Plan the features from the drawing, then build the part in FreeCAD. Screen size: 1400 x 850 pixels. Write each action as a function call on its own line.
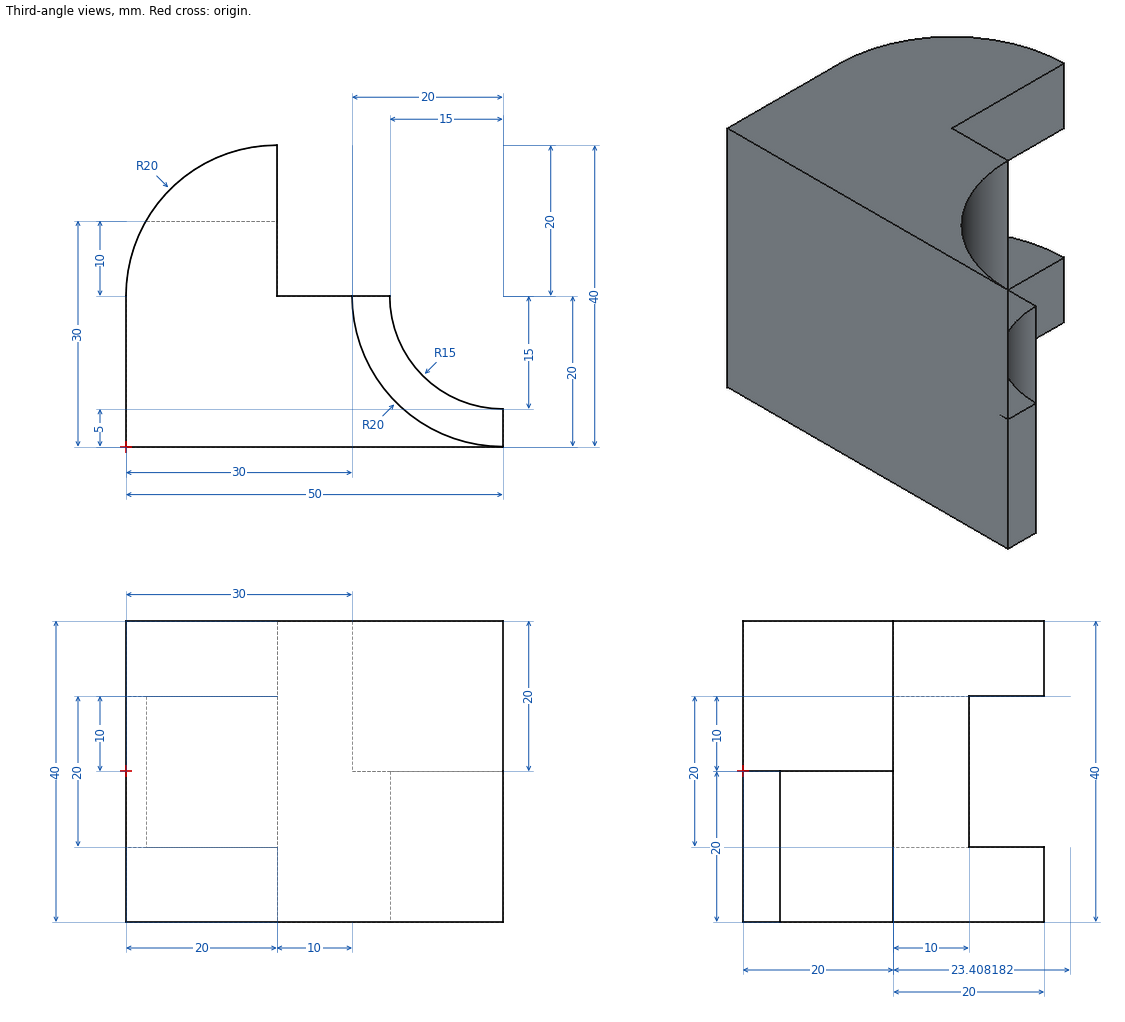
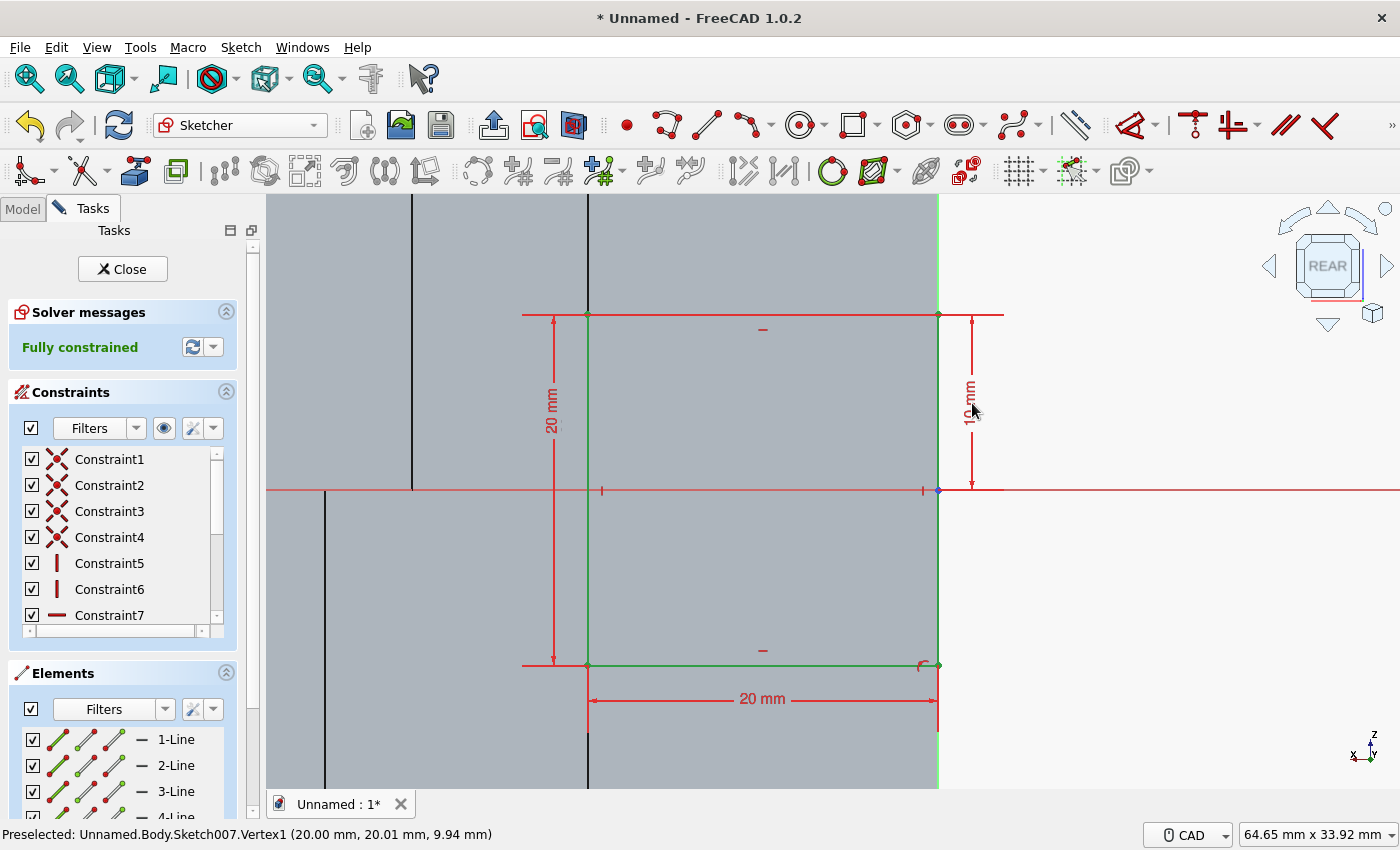
click(123, 269)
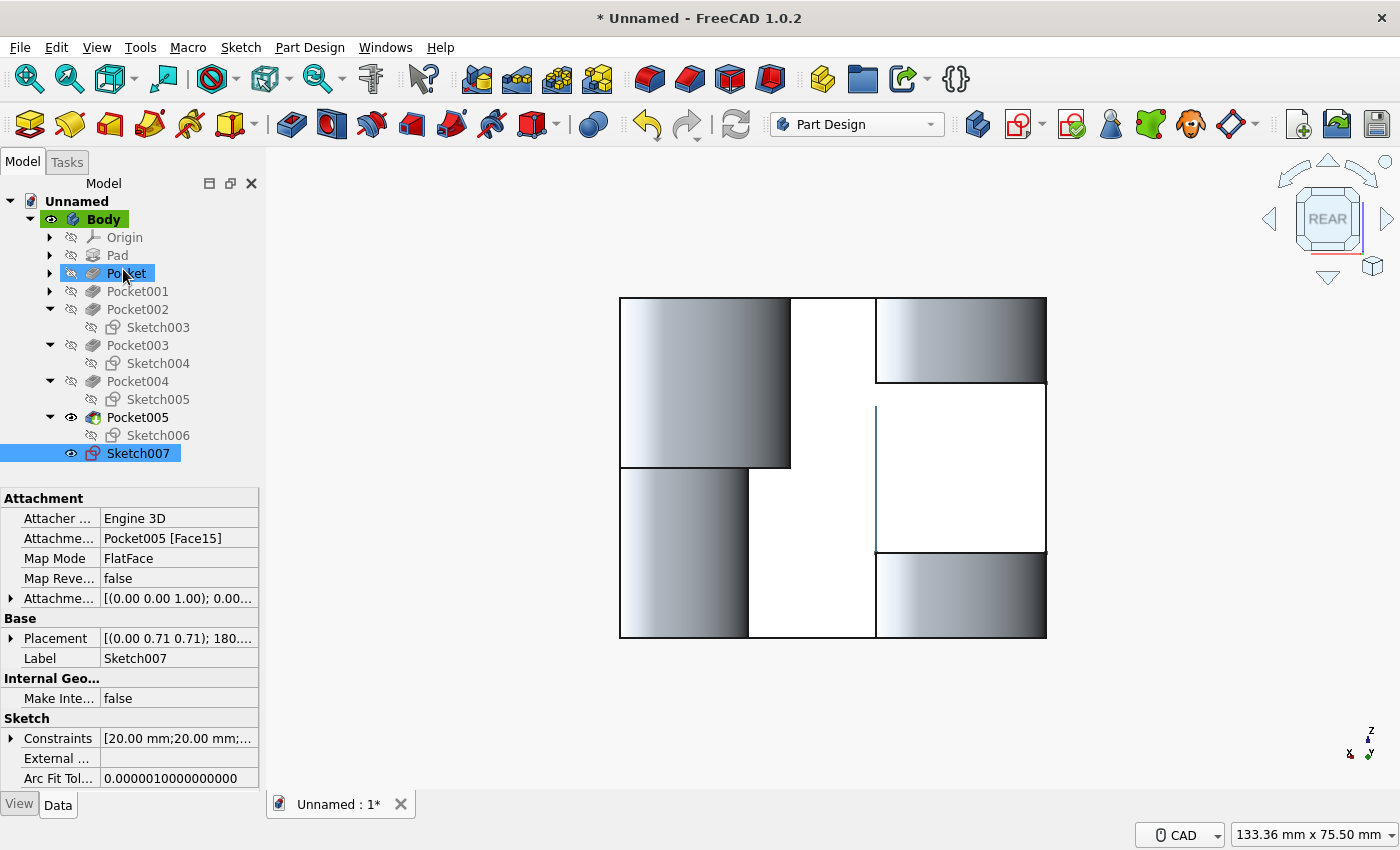
click(30, 124)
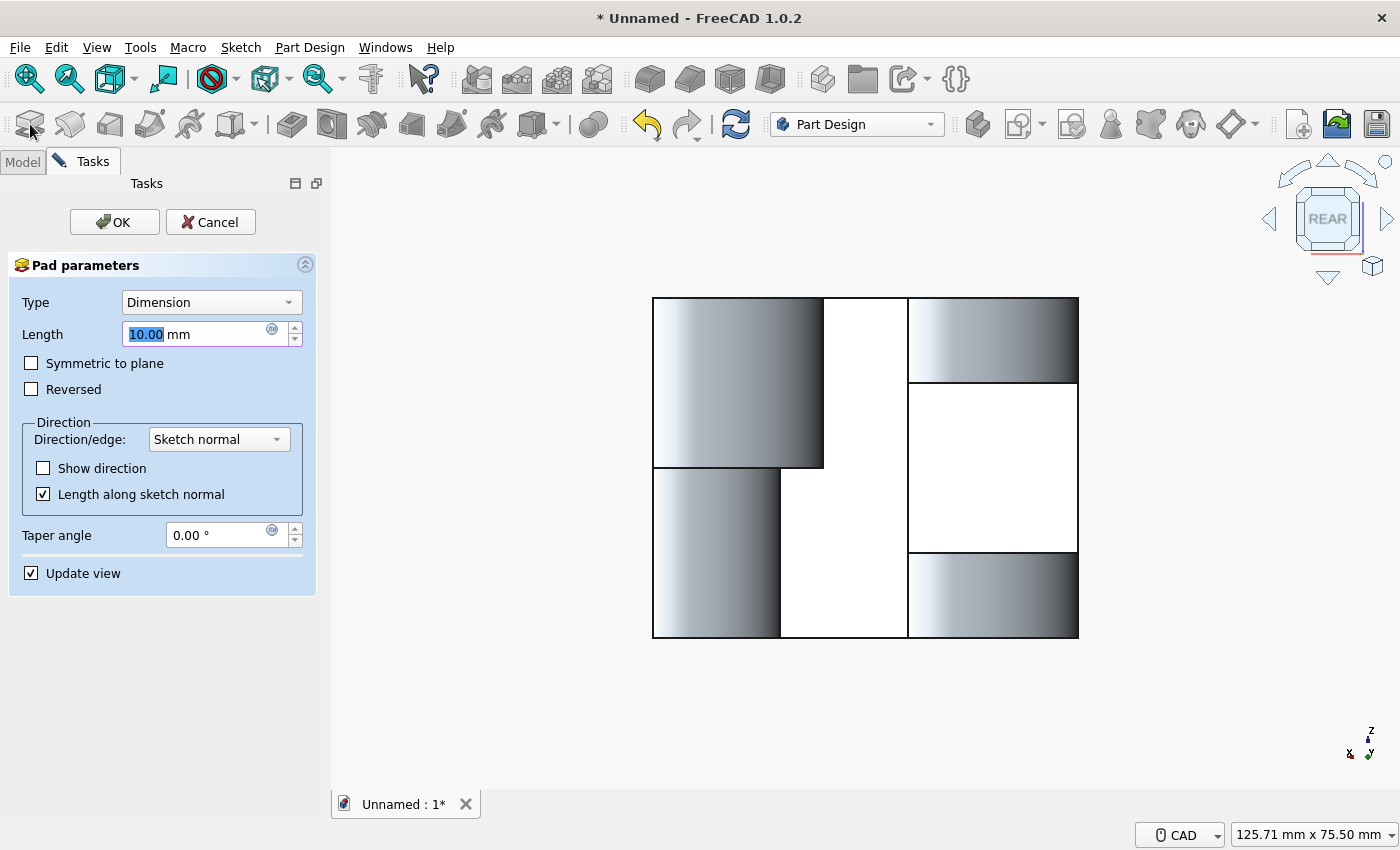
text(10)
key(Tab)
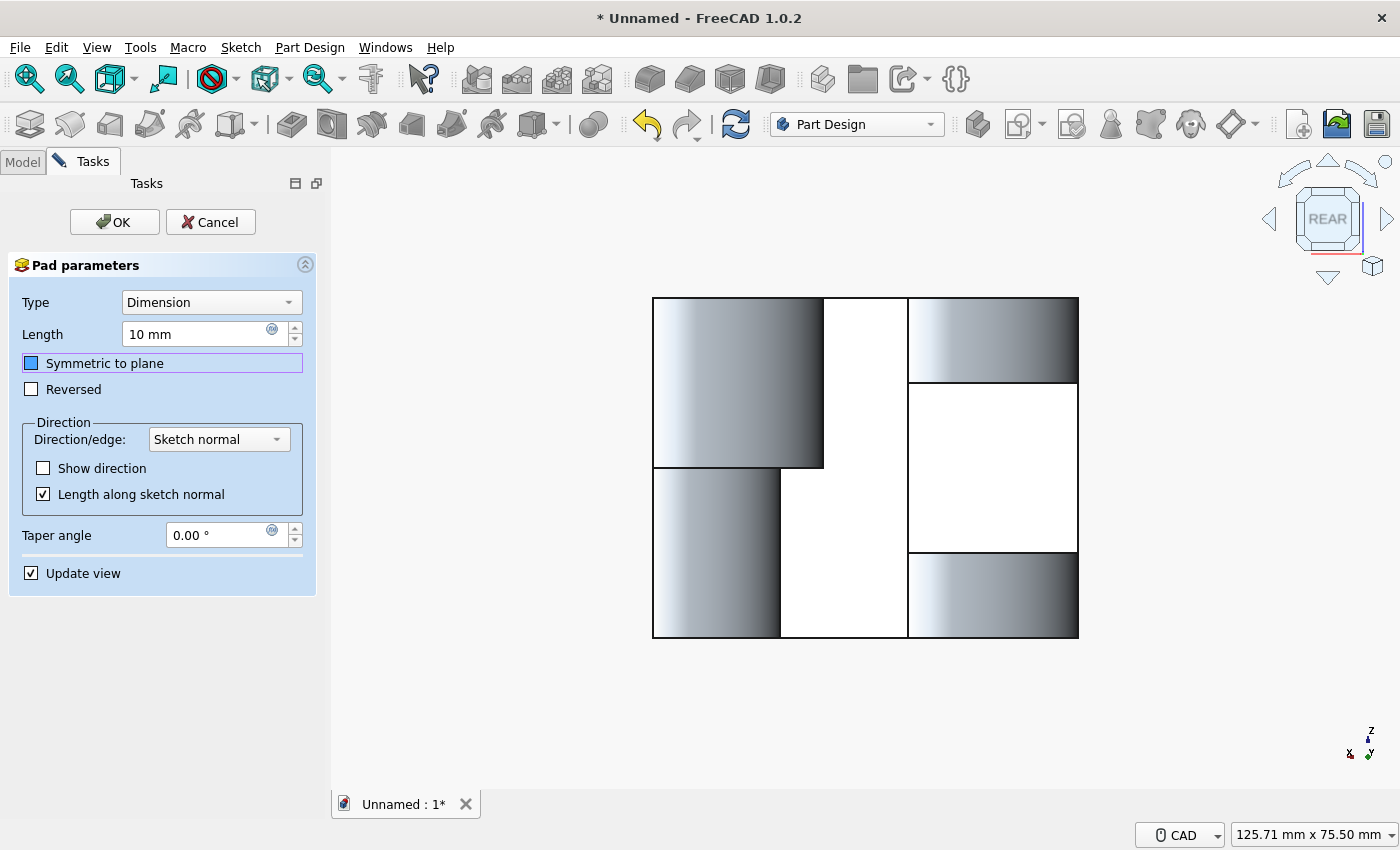
click(115, 222)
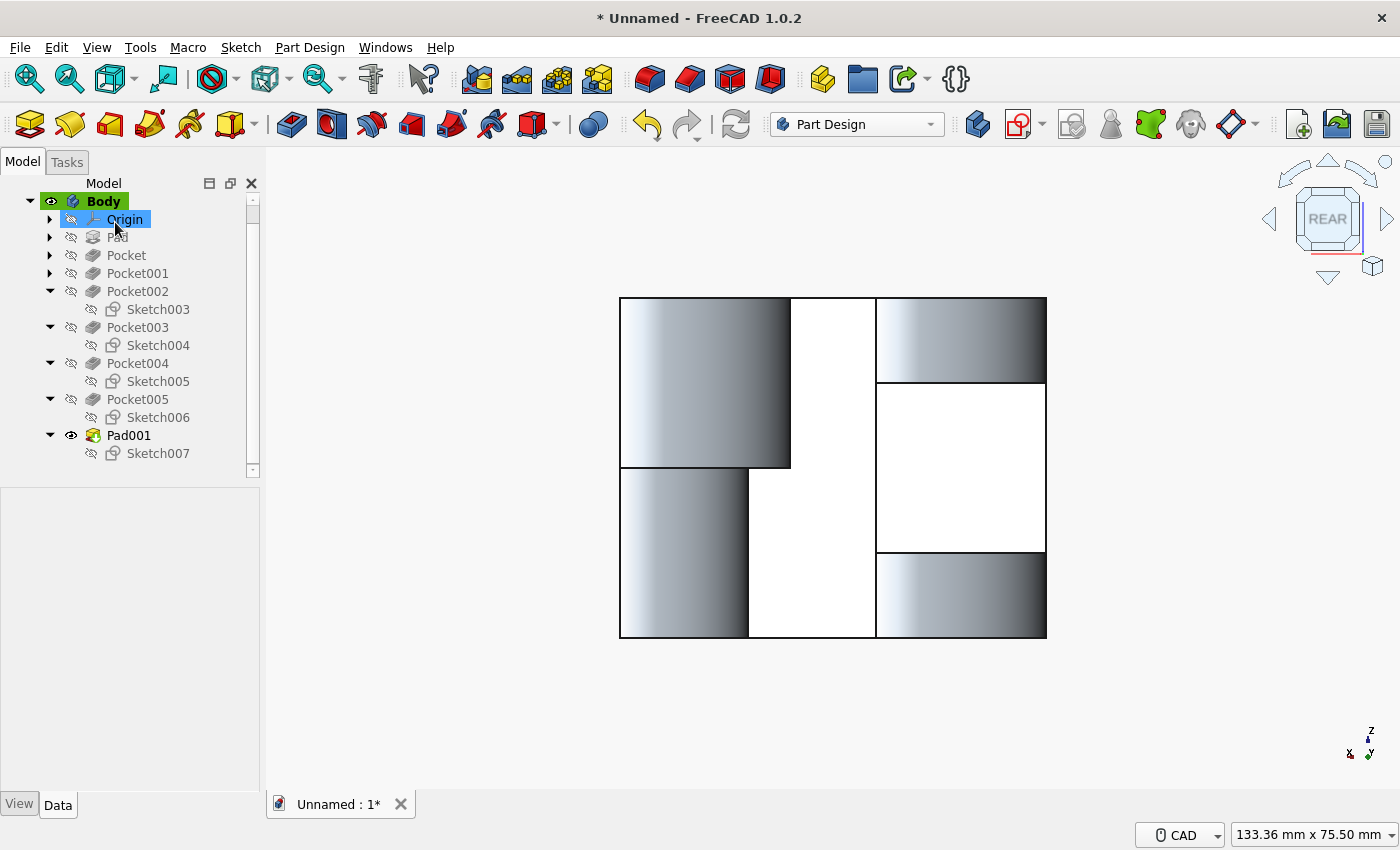
key(0)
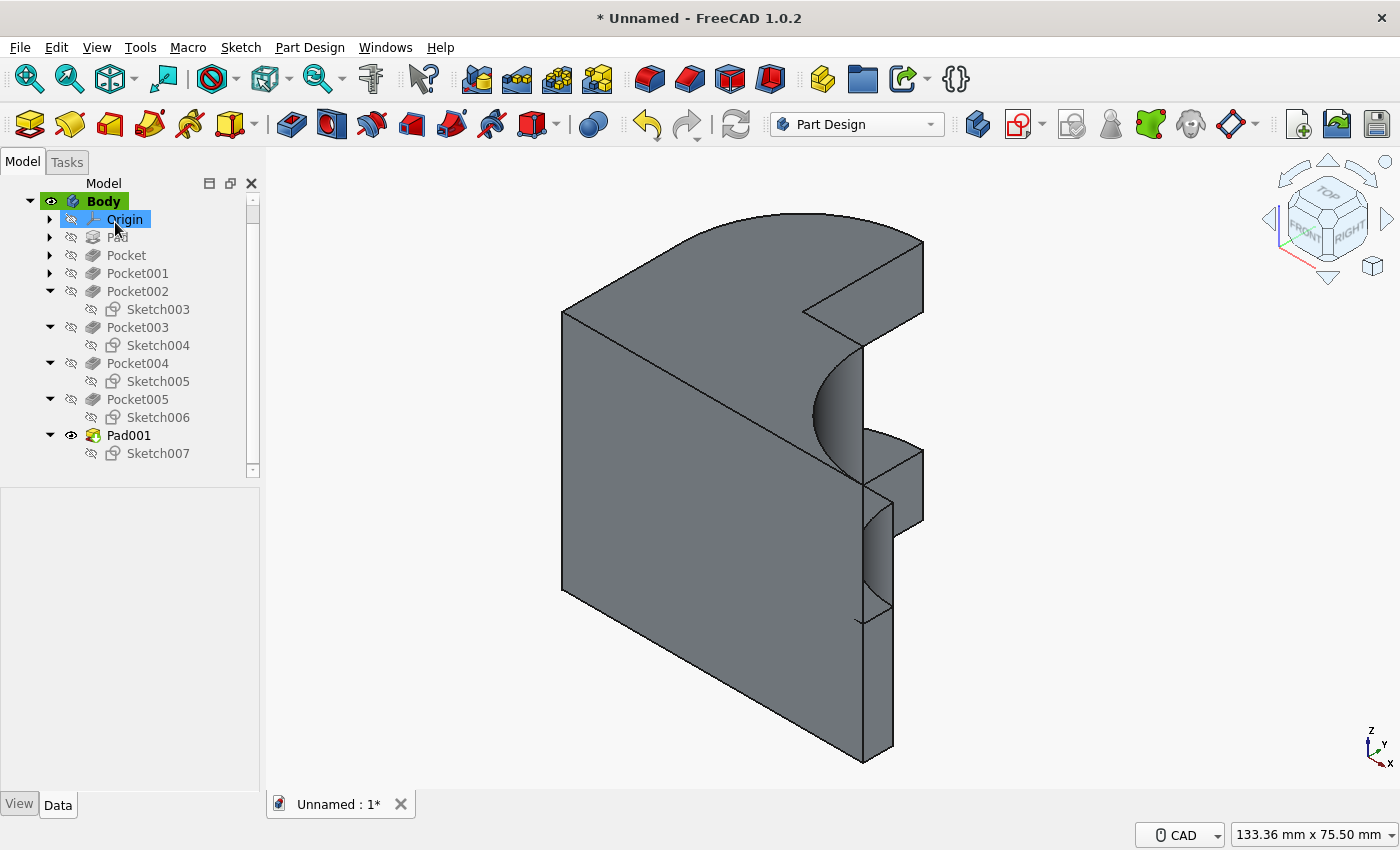
scroll(747, 283, up, 4)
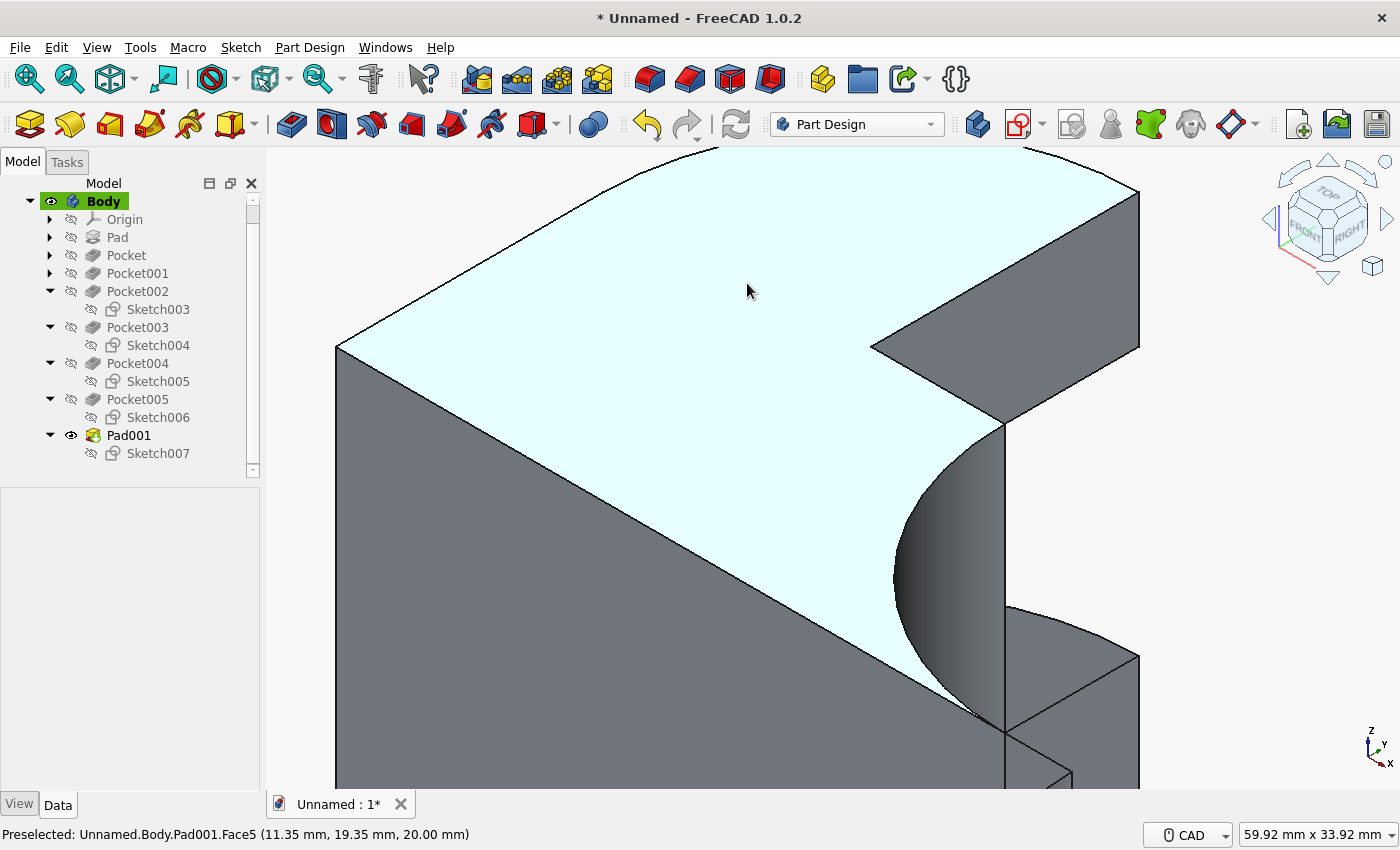
click(30, 80)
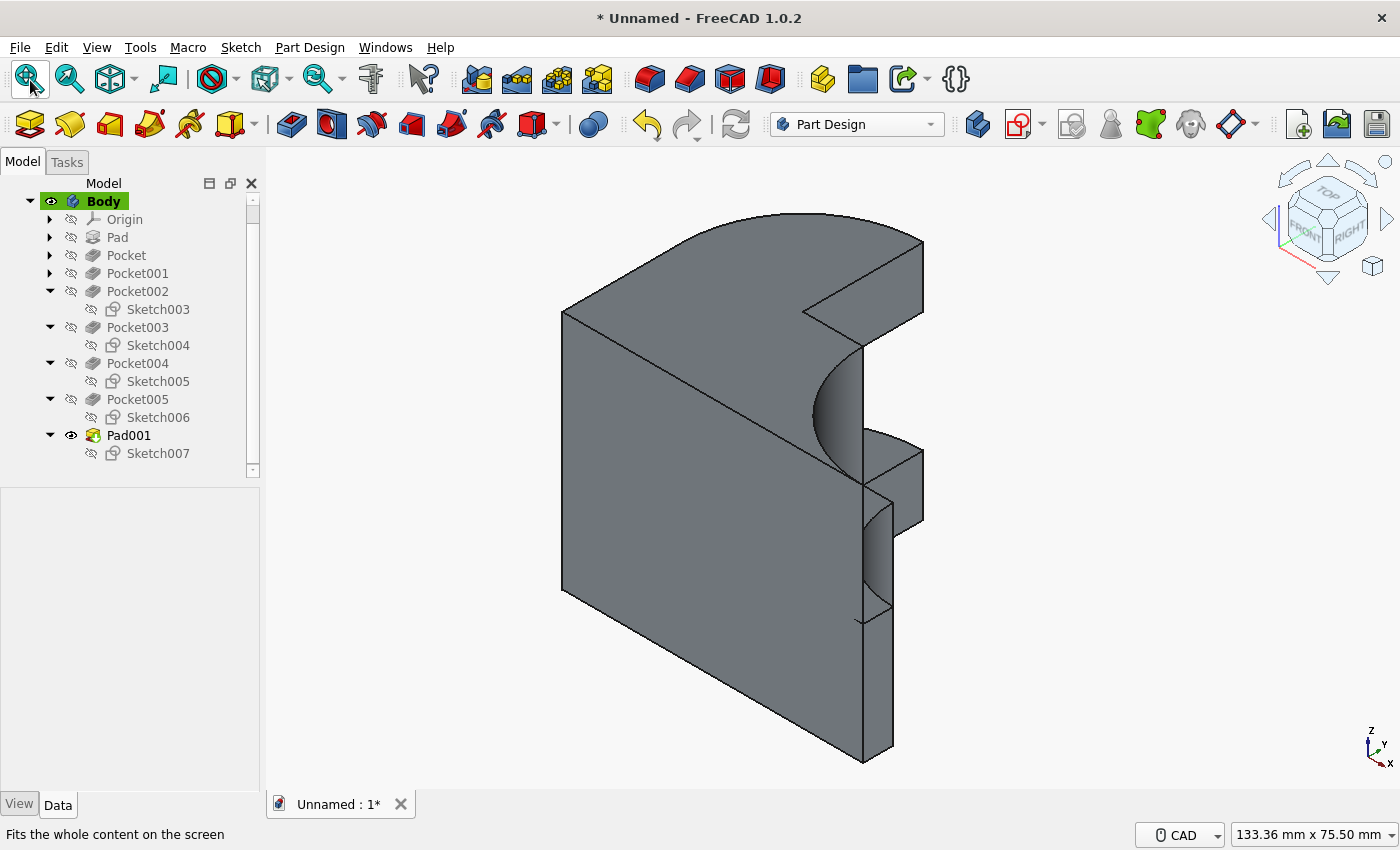
key(2)